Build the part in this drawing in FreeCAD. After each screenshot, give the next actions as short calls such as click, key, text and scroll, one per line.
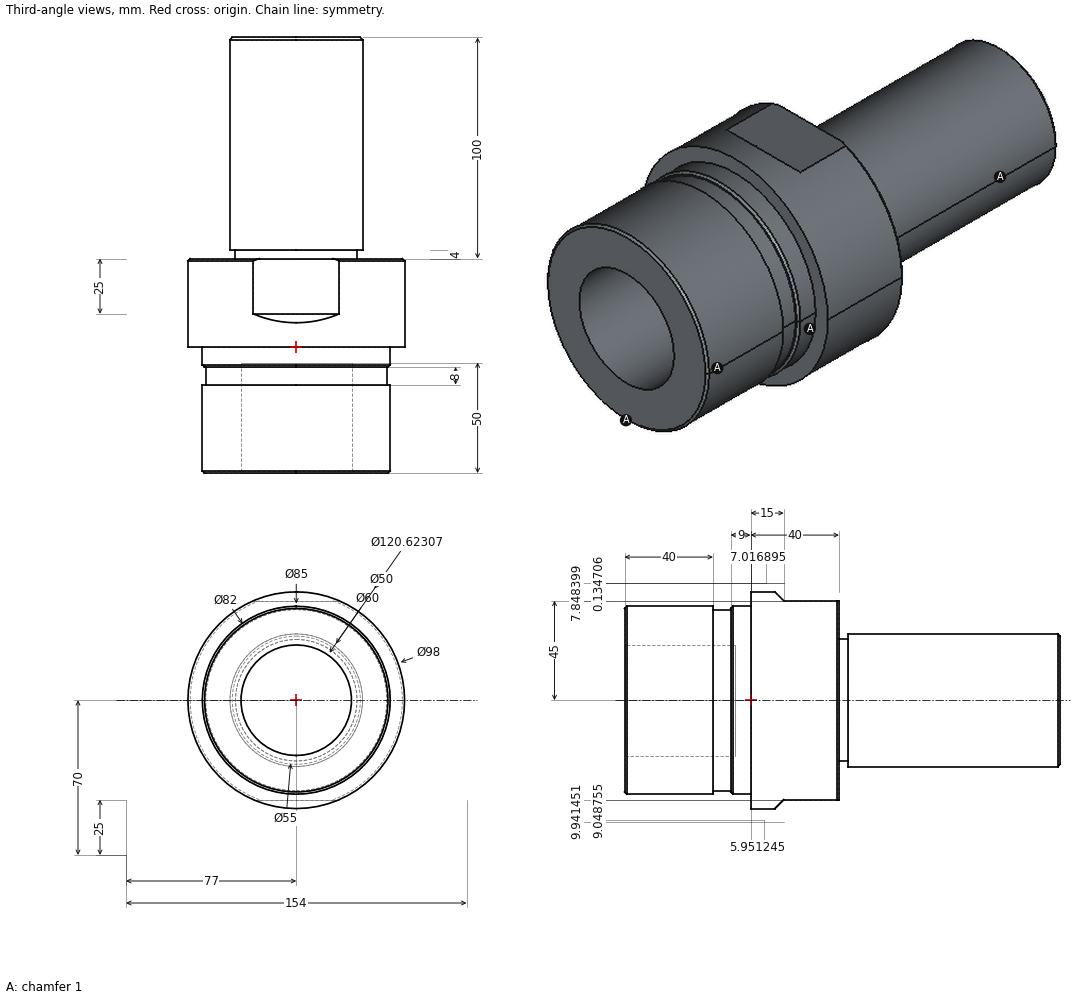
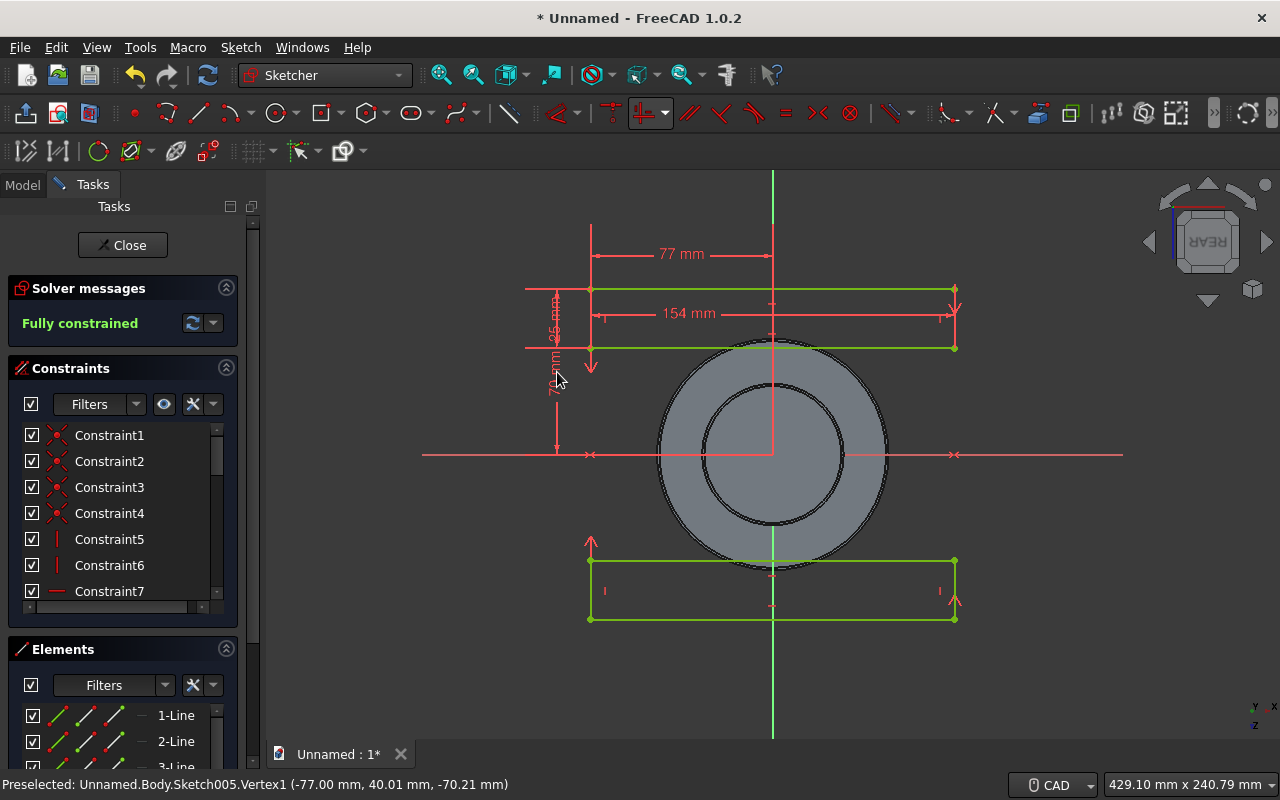
click(123, 245)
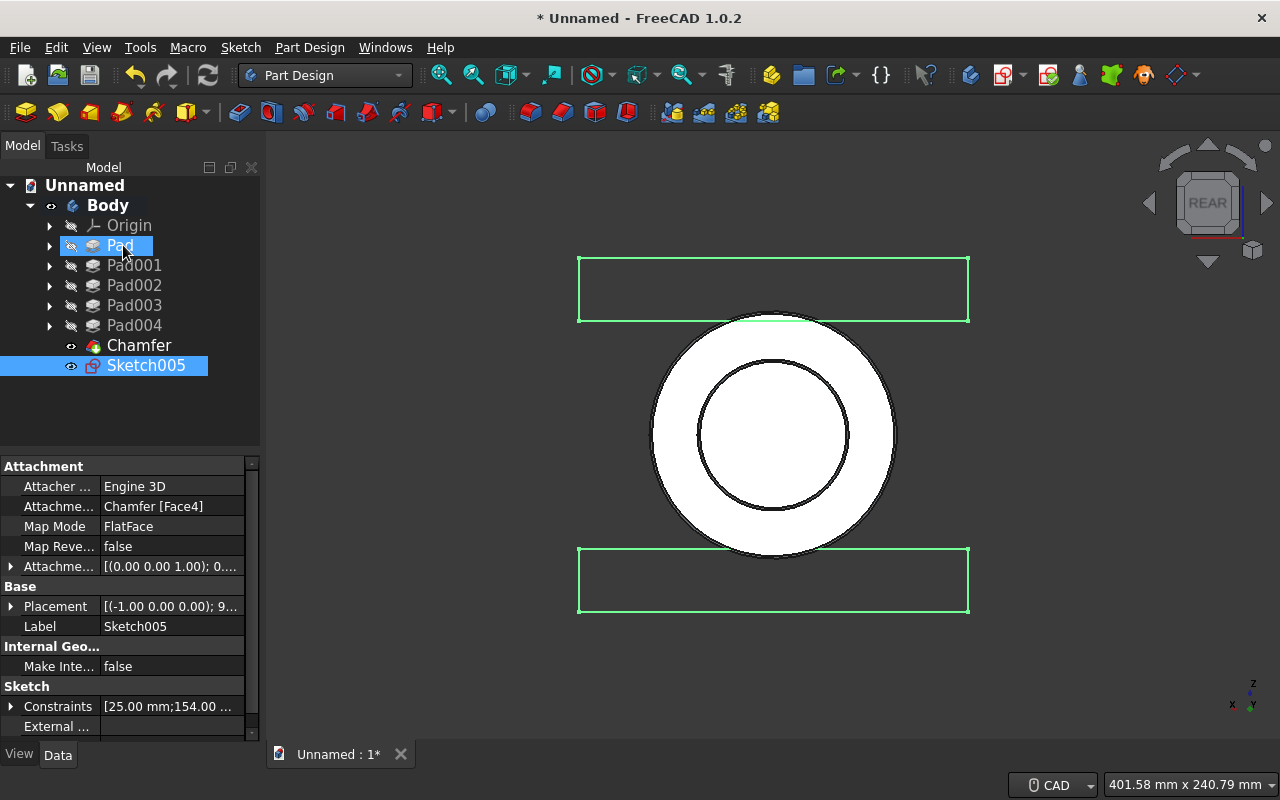
click(240, 112)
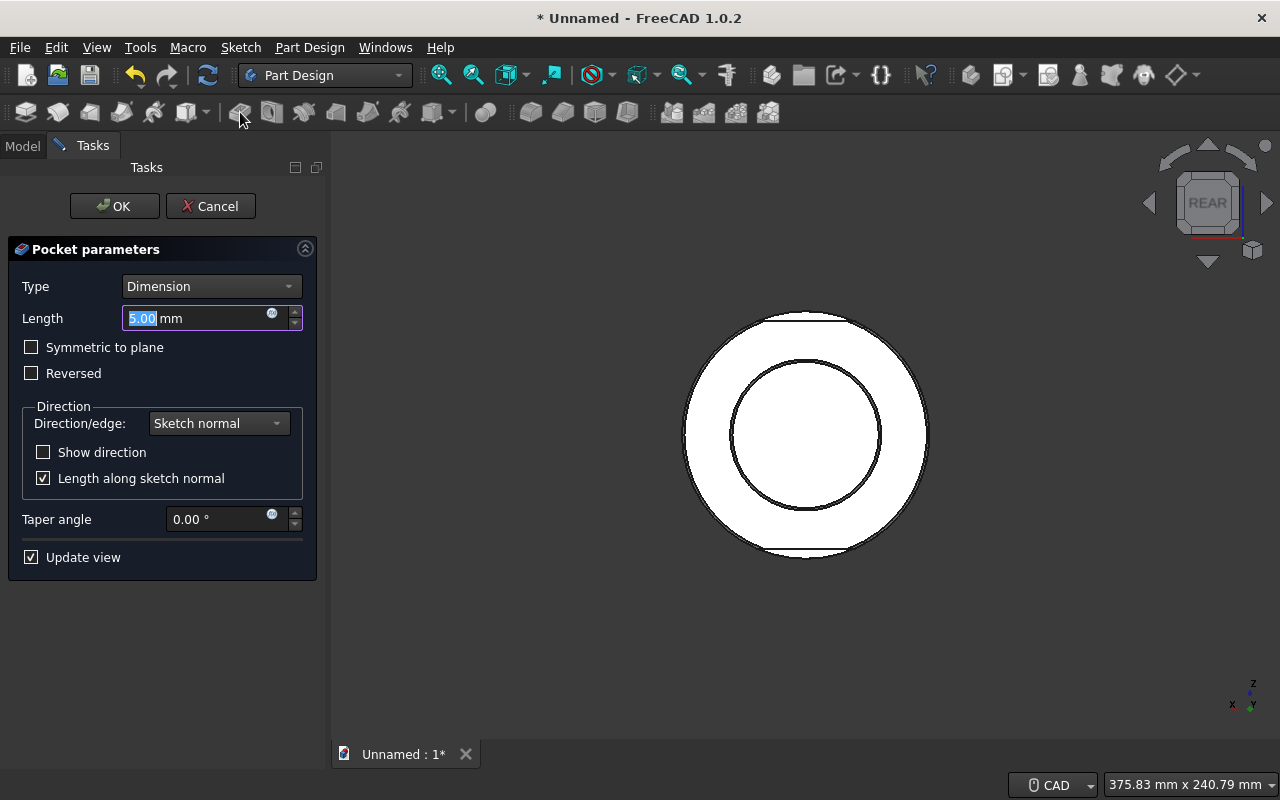
text(25)
key(Tab)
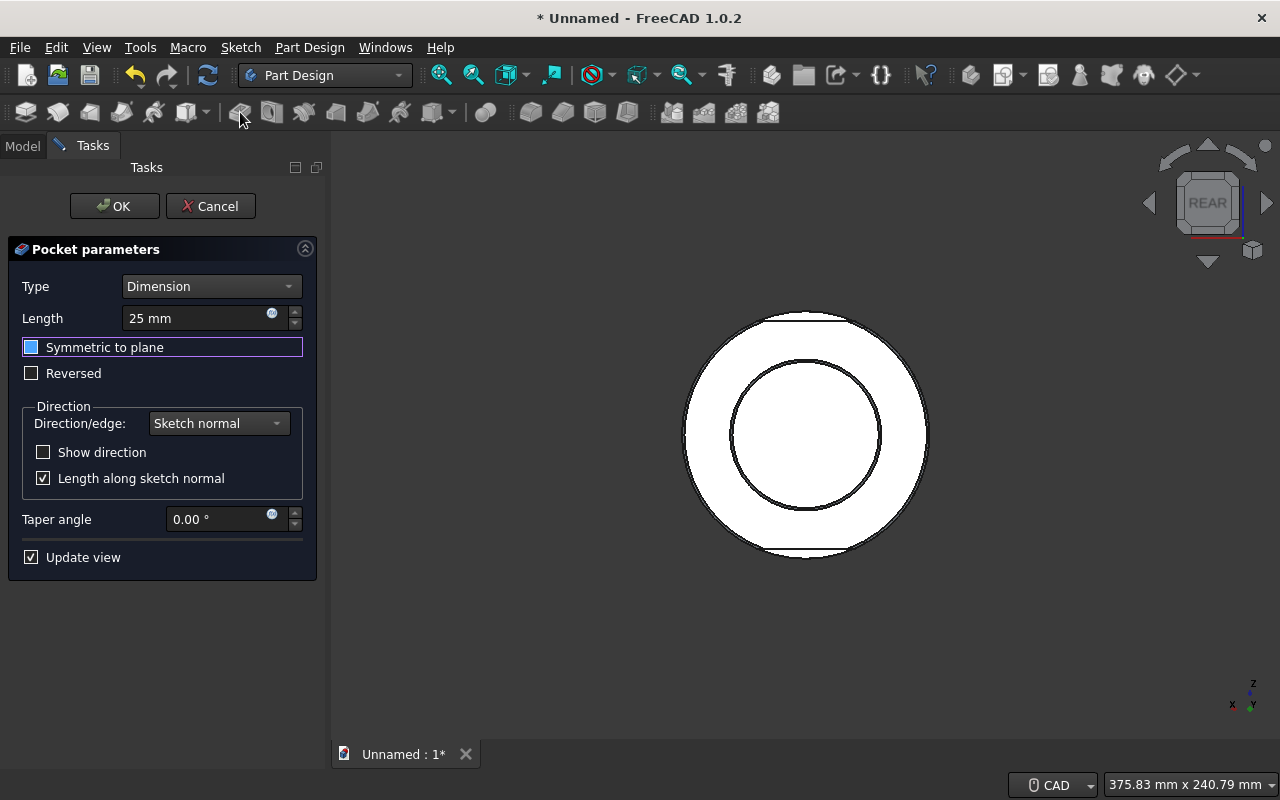
click(115, 206)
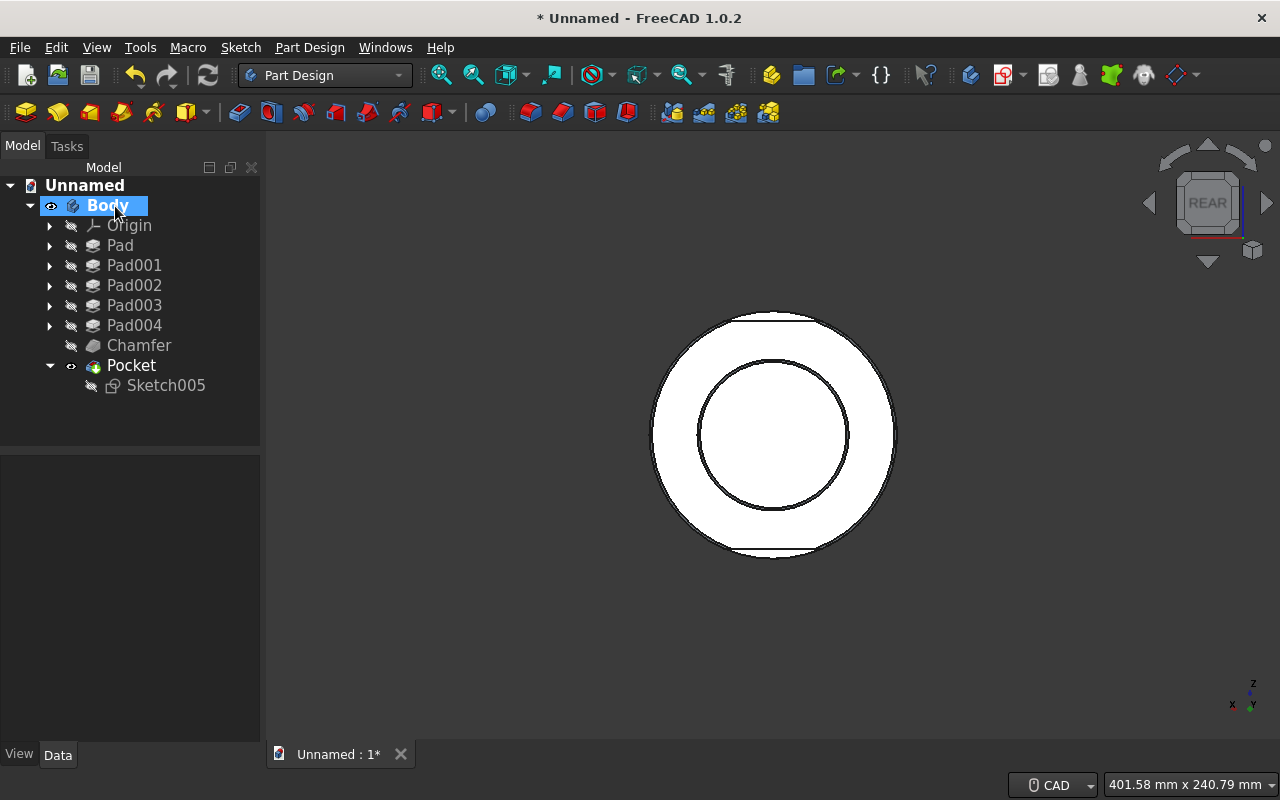
click(442, 76)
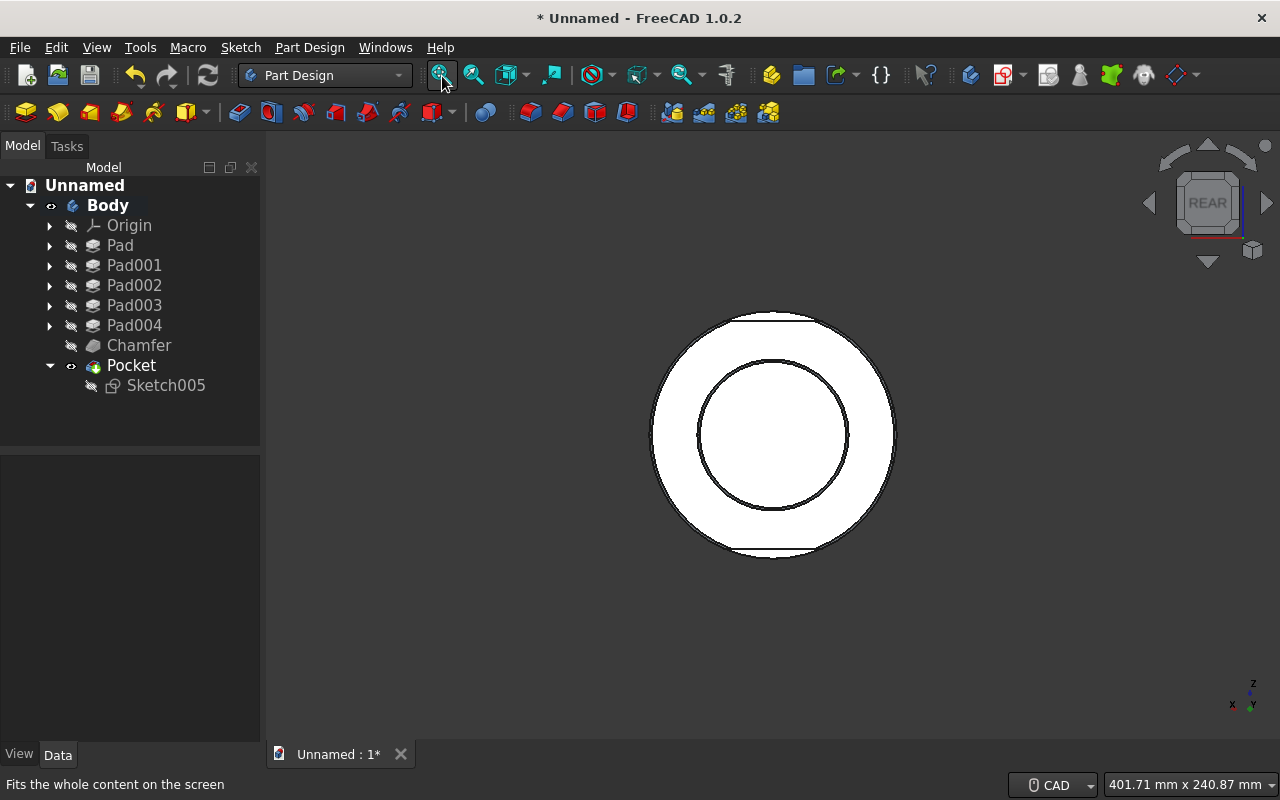
click(1004, 76)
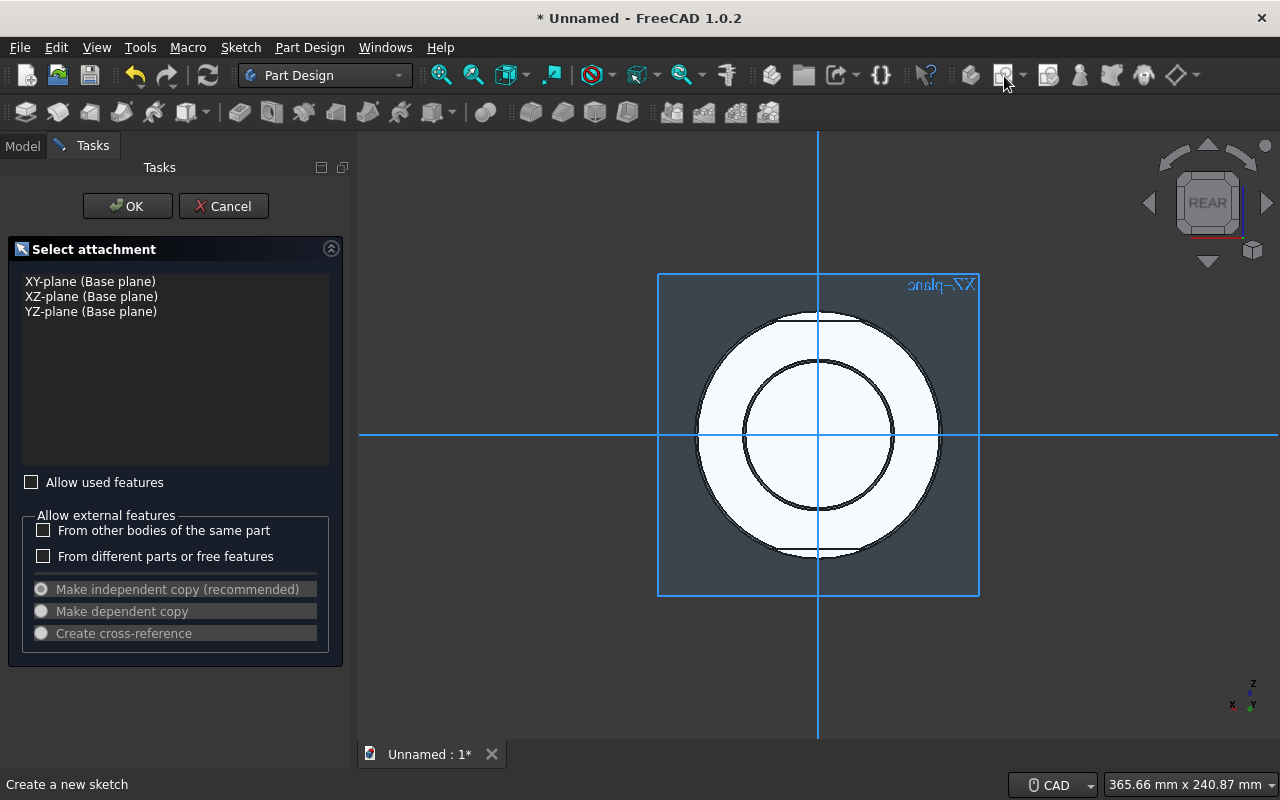
click(82, 312)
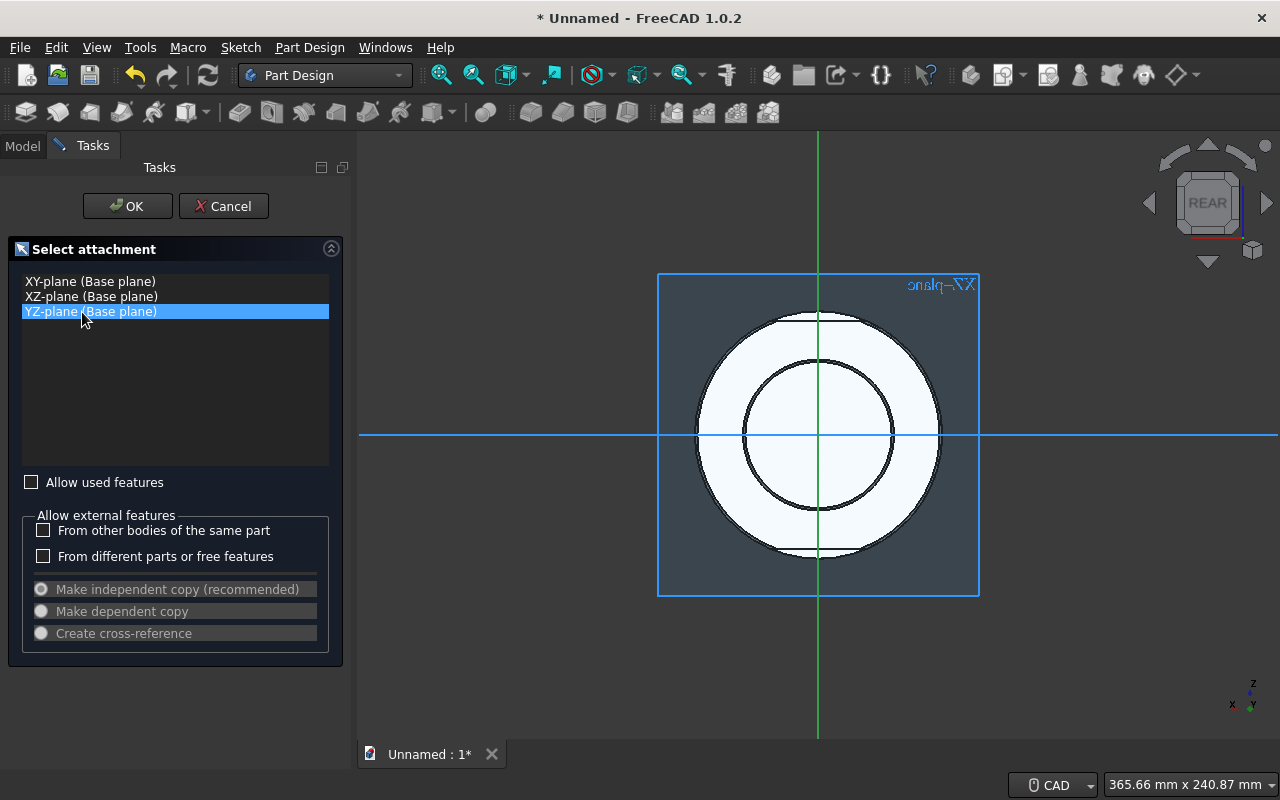
click(128, 206)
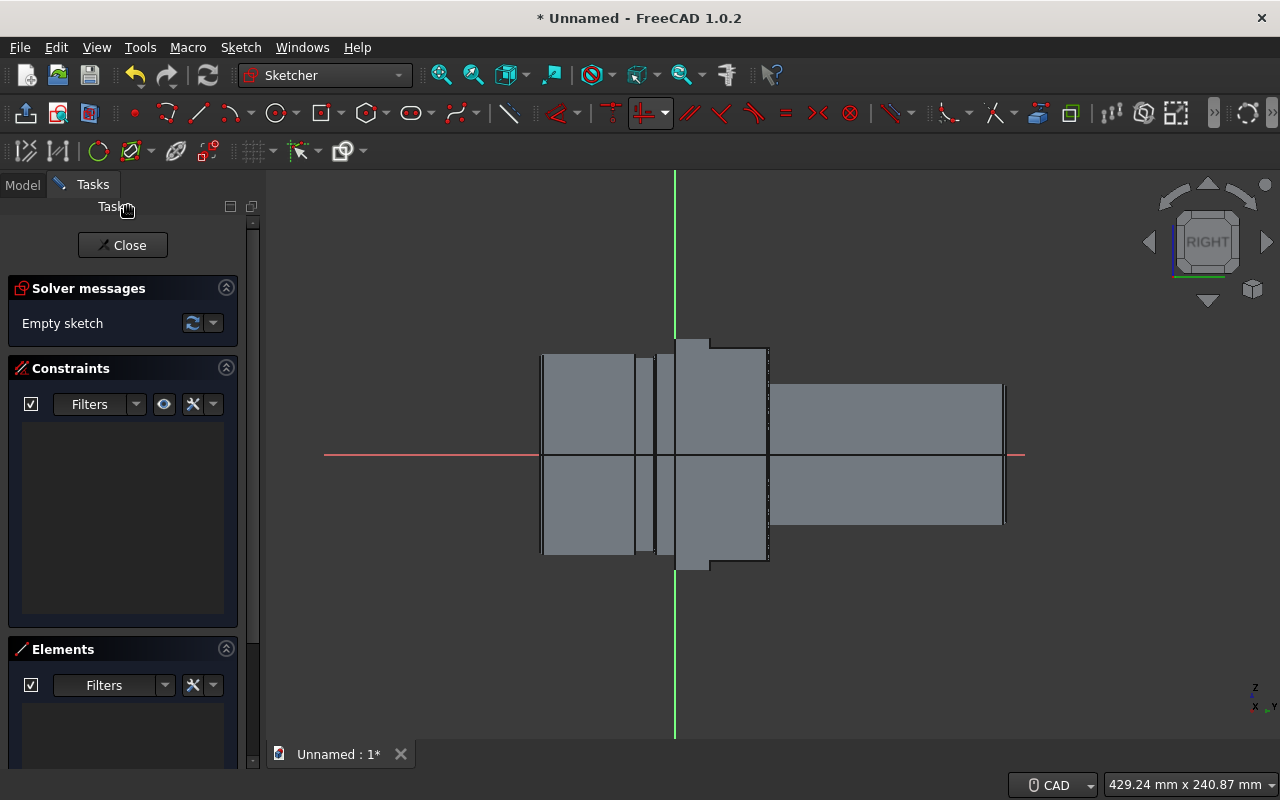
click(90, 114)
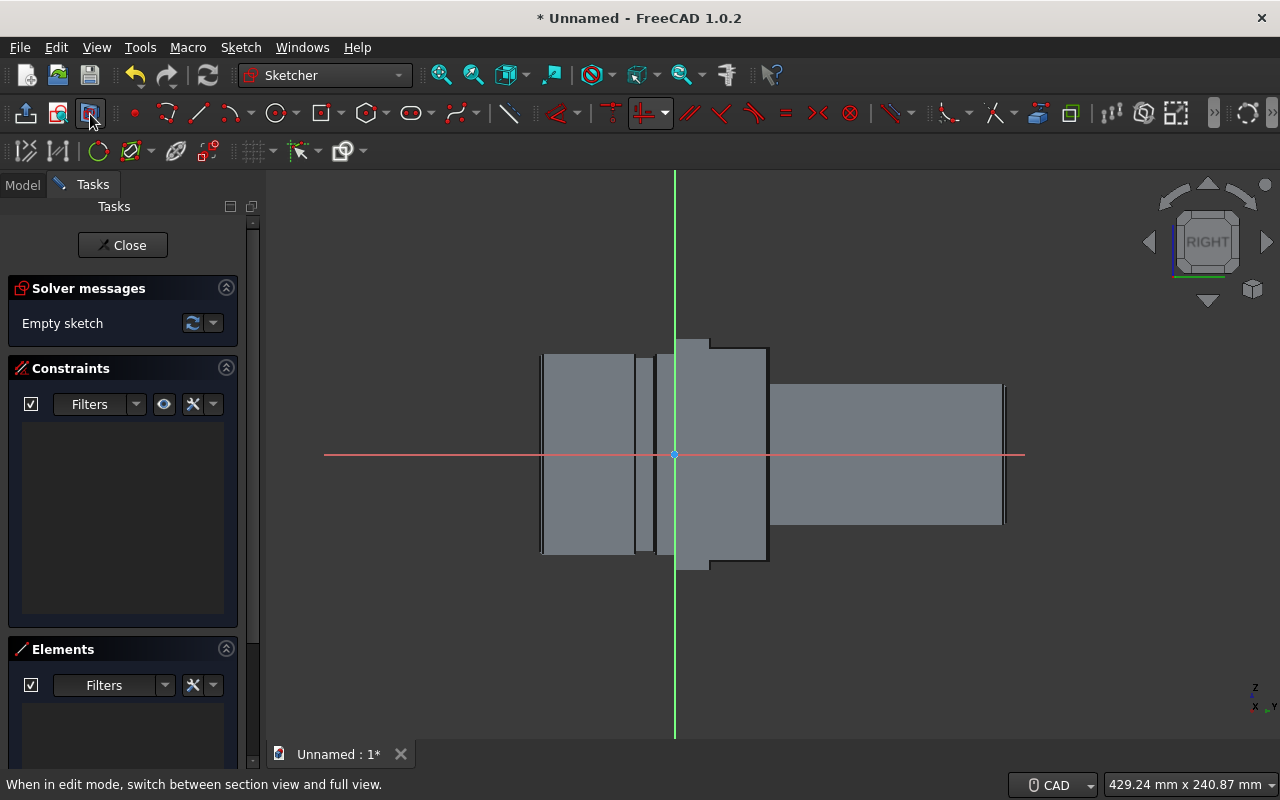
scroll(669, 462, up, 2)